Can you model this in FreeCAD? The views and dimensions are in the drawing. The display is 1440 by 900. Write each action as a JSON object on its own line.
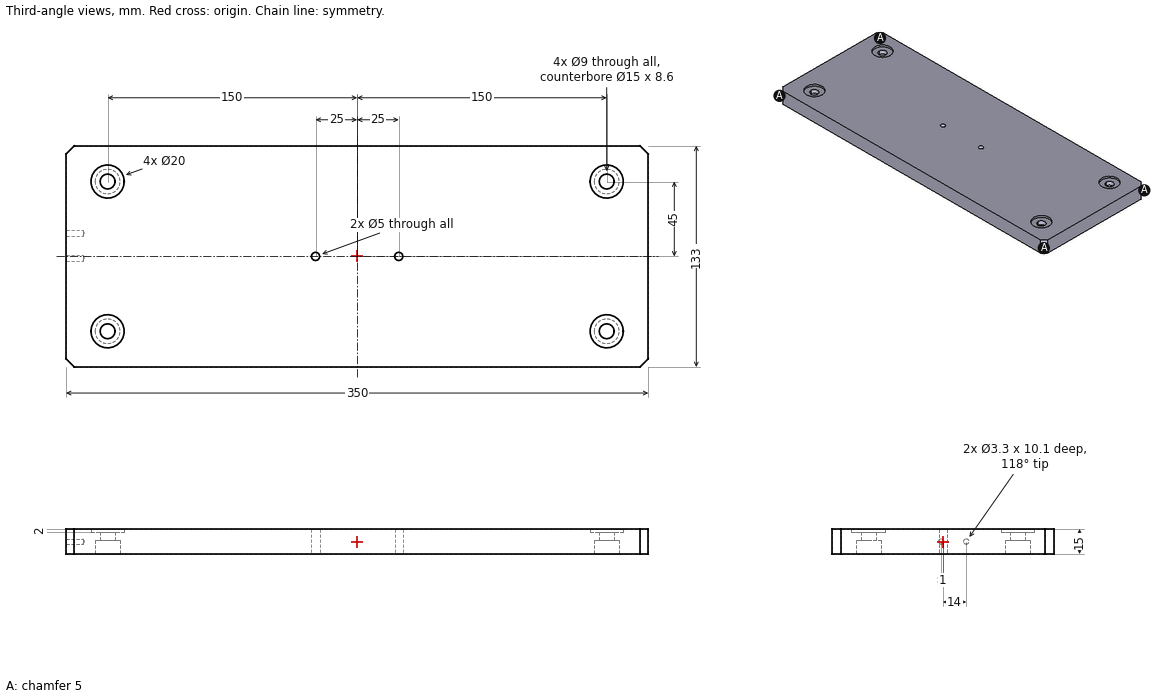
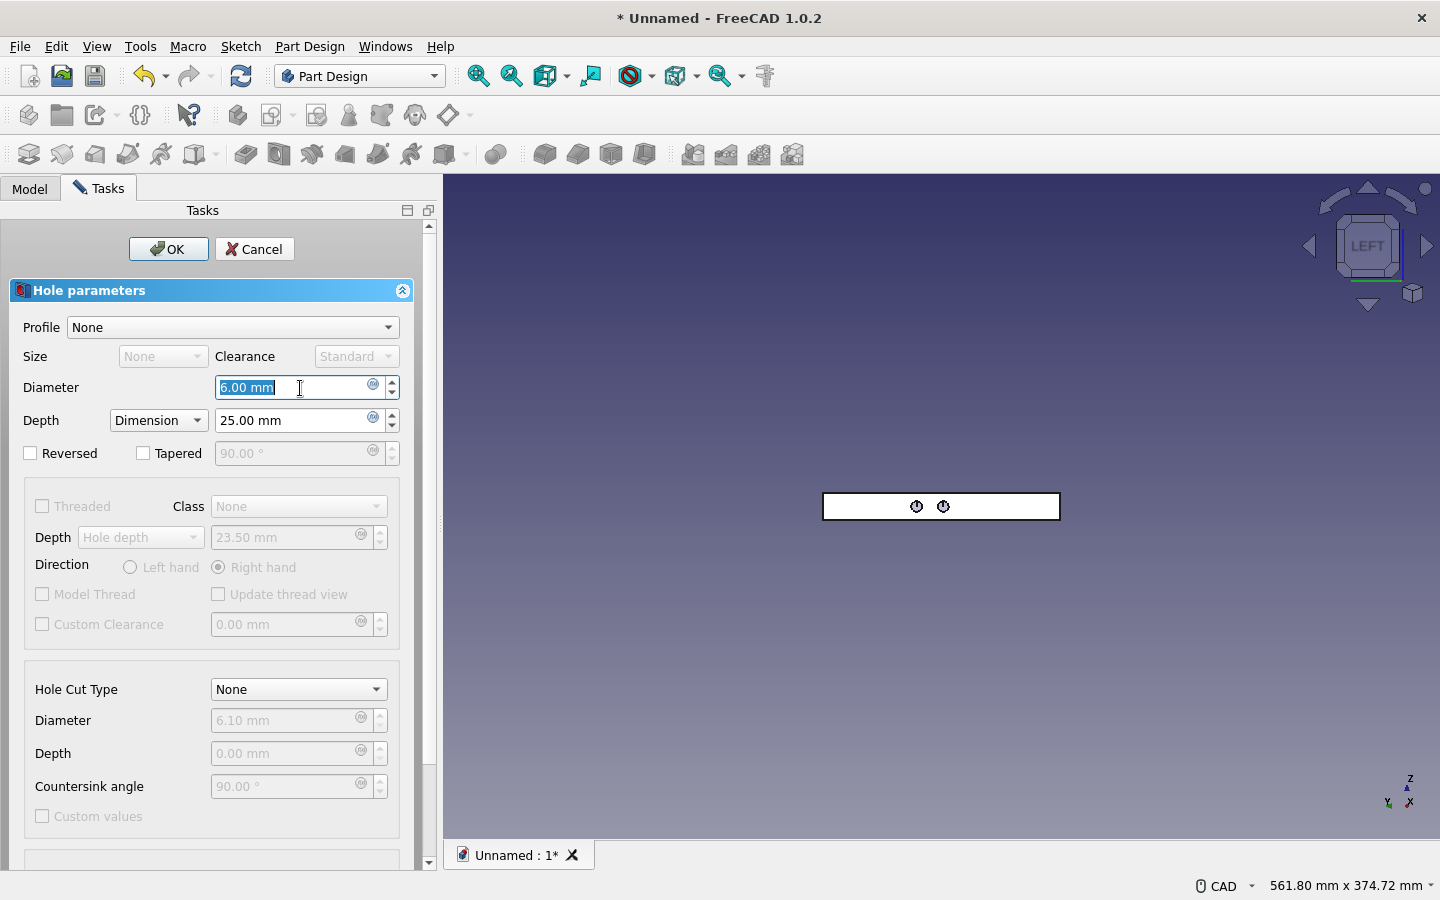
{"action": "type", "text": "3.3"}
{"action": "key", "text": "Tab"}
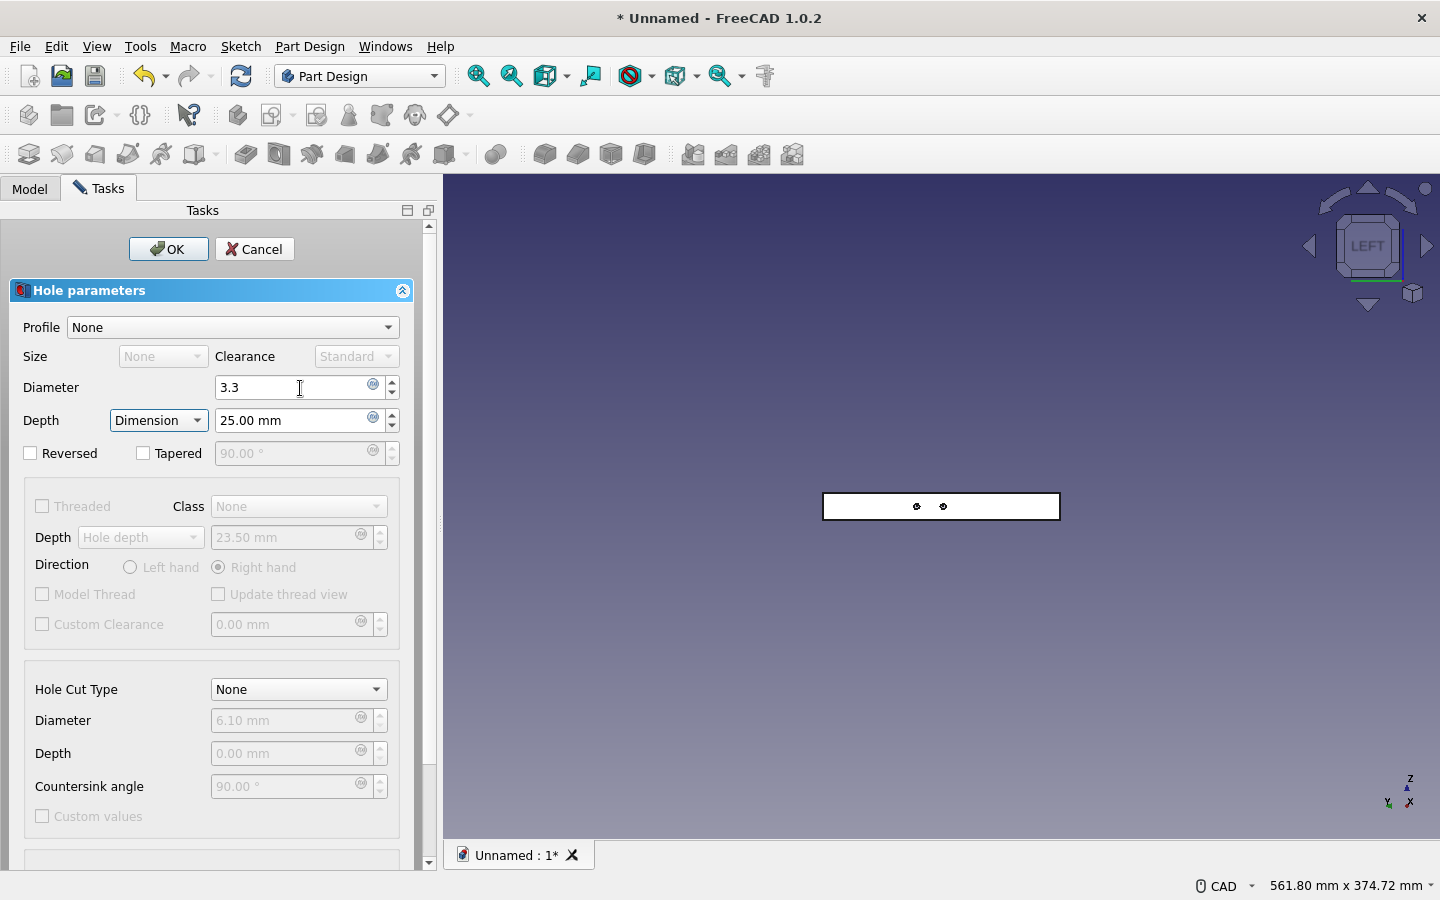
{"action": "triple_click", "coordinate": [300, 420]}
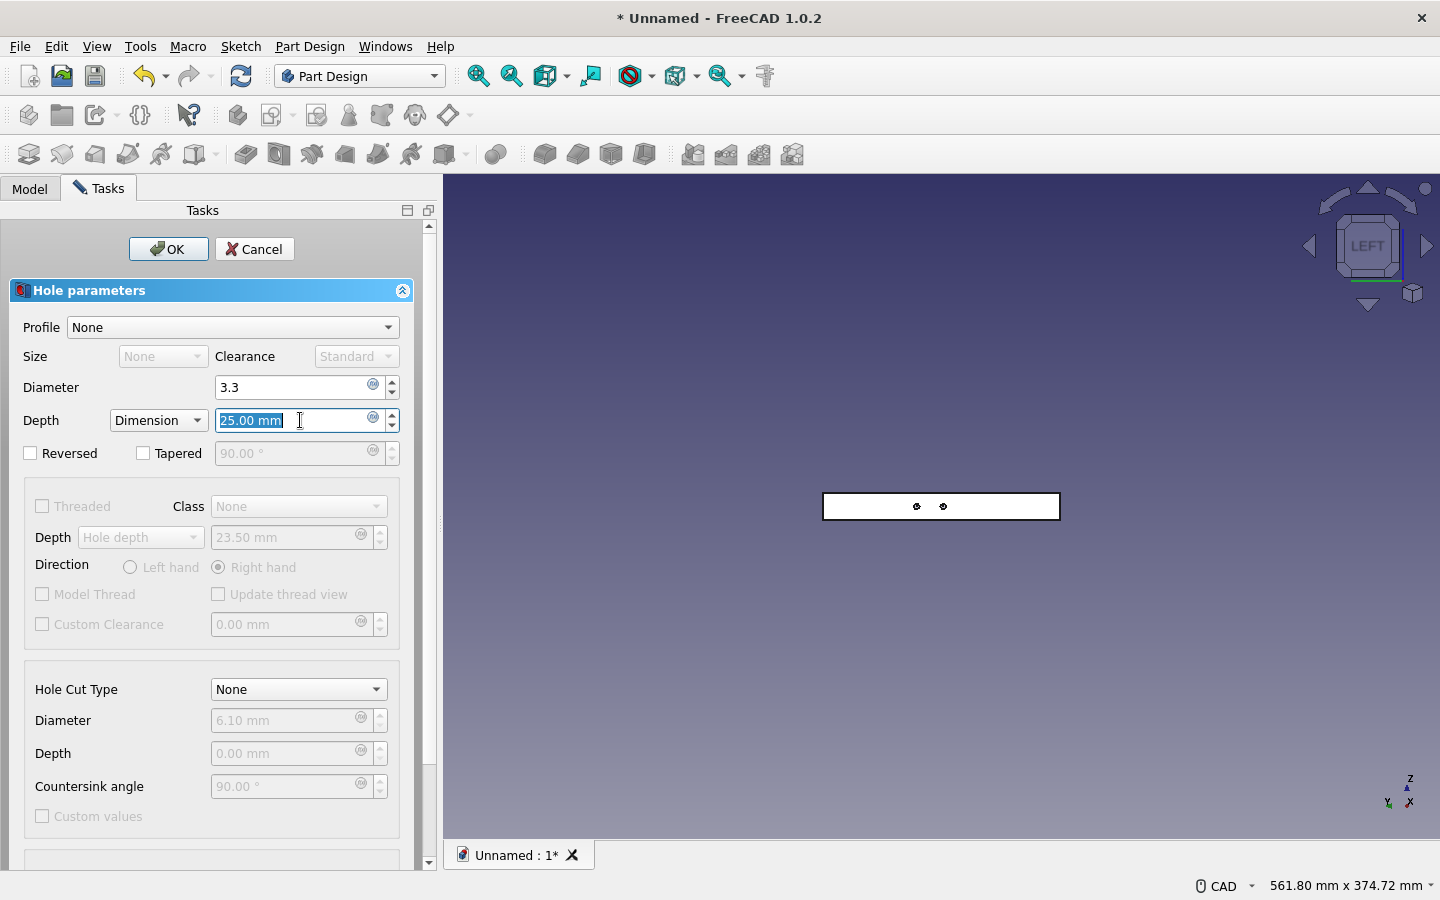
{"action": "type", "text": "10.1"}
{"action": "key", "text": "Tab"}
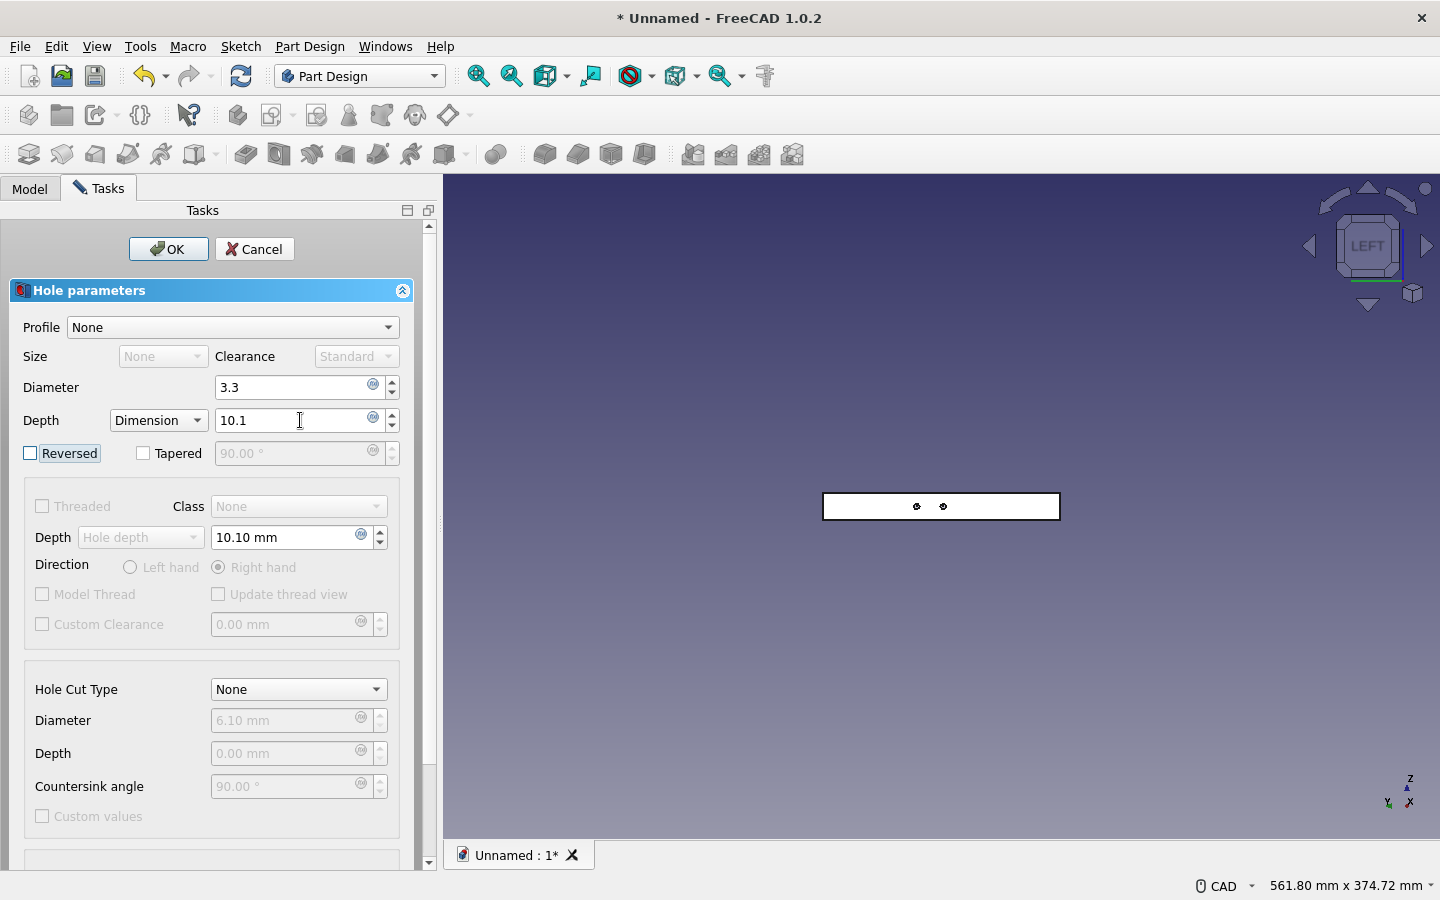
{"action": "left_click", "coordinate": [169, 249]}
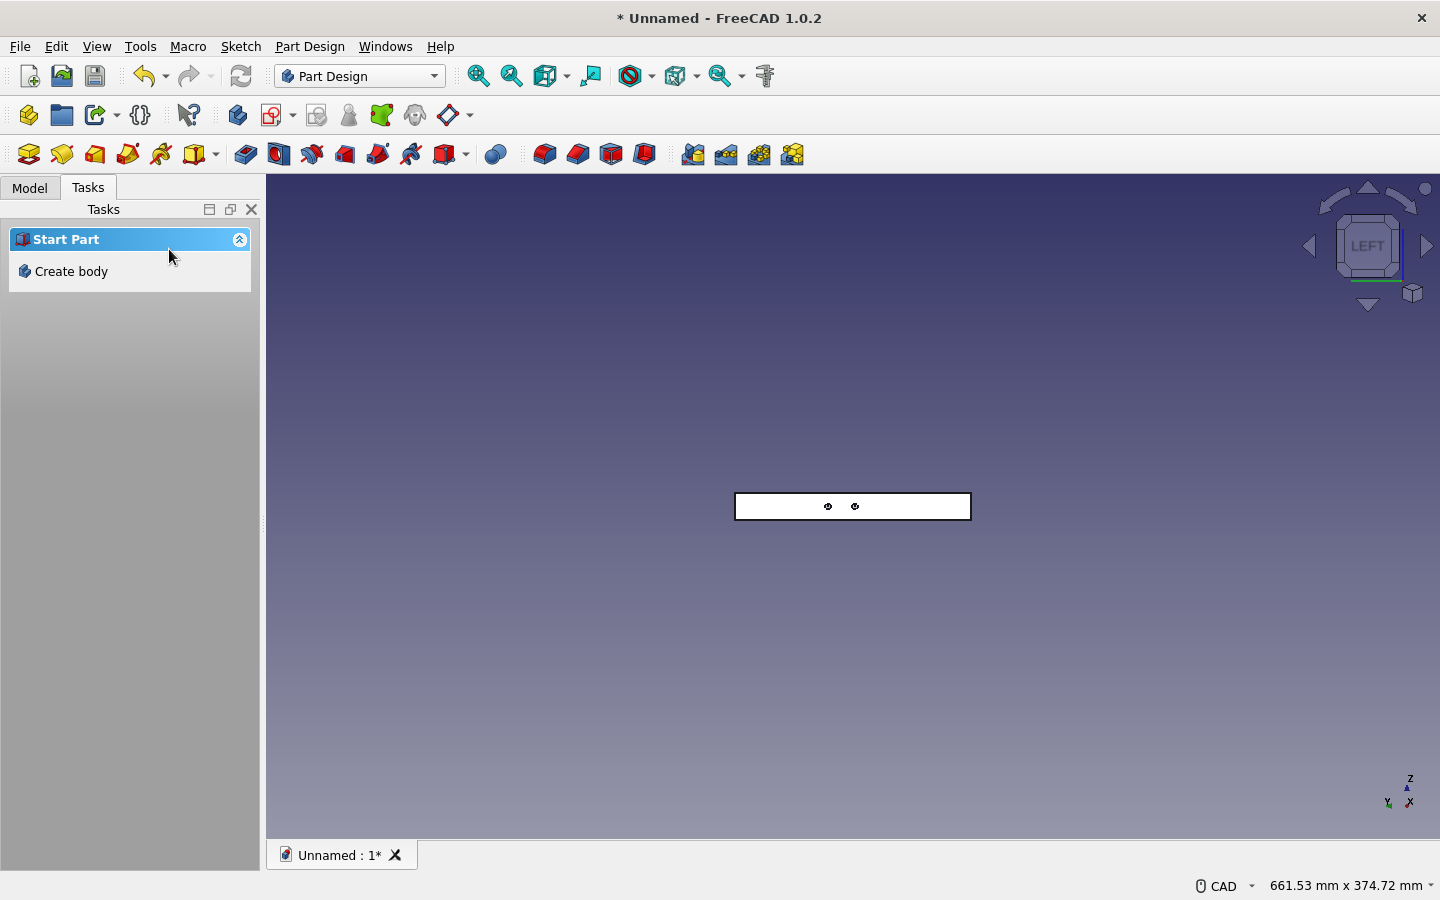
{"action": "key", "text": "v f"}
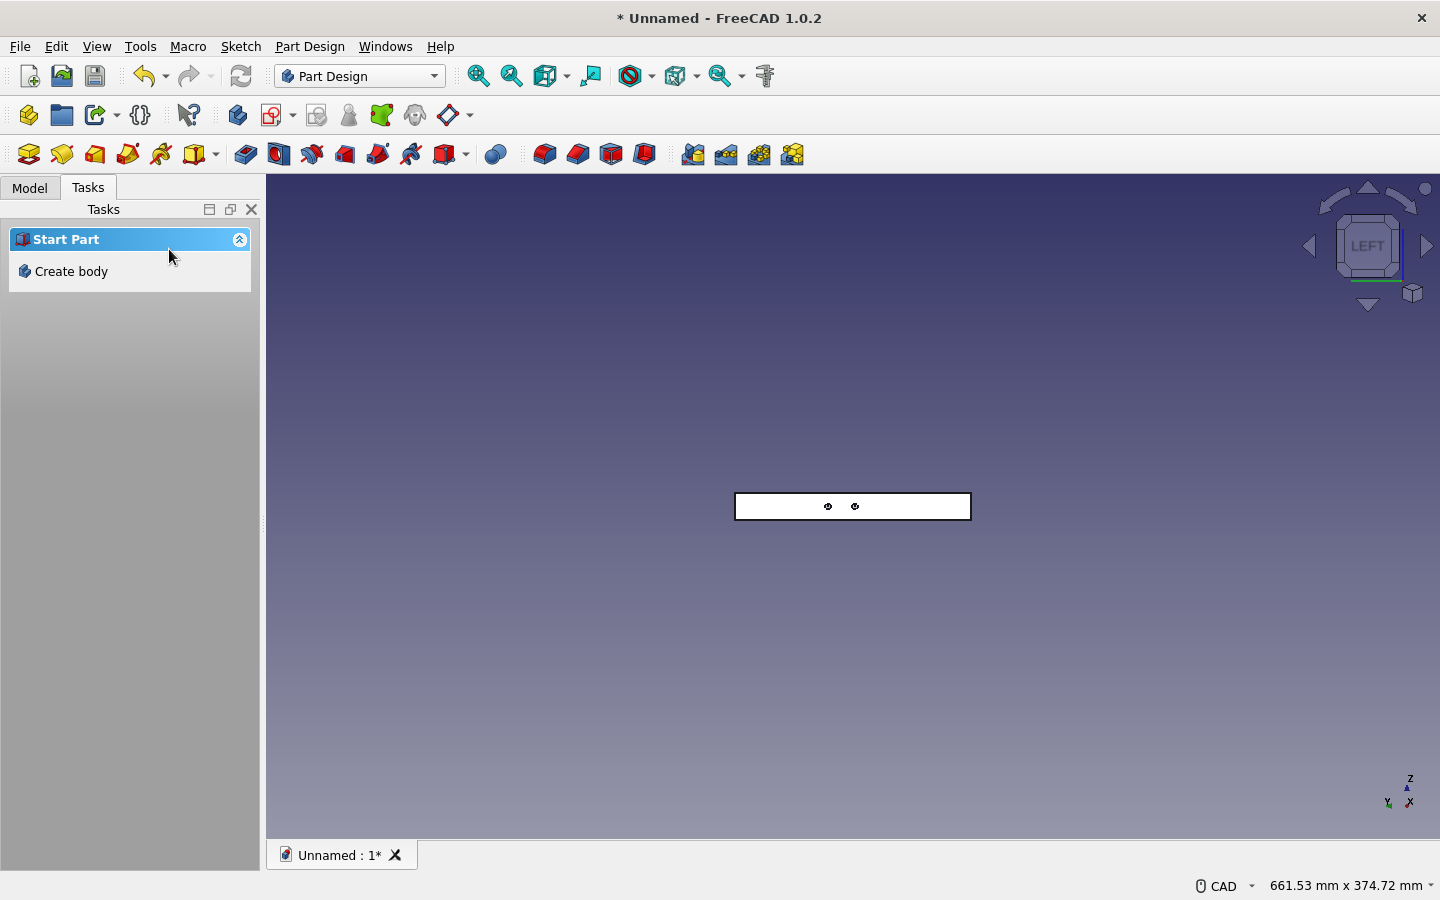
{"action": "left_click", "coordinate": [971, 505]}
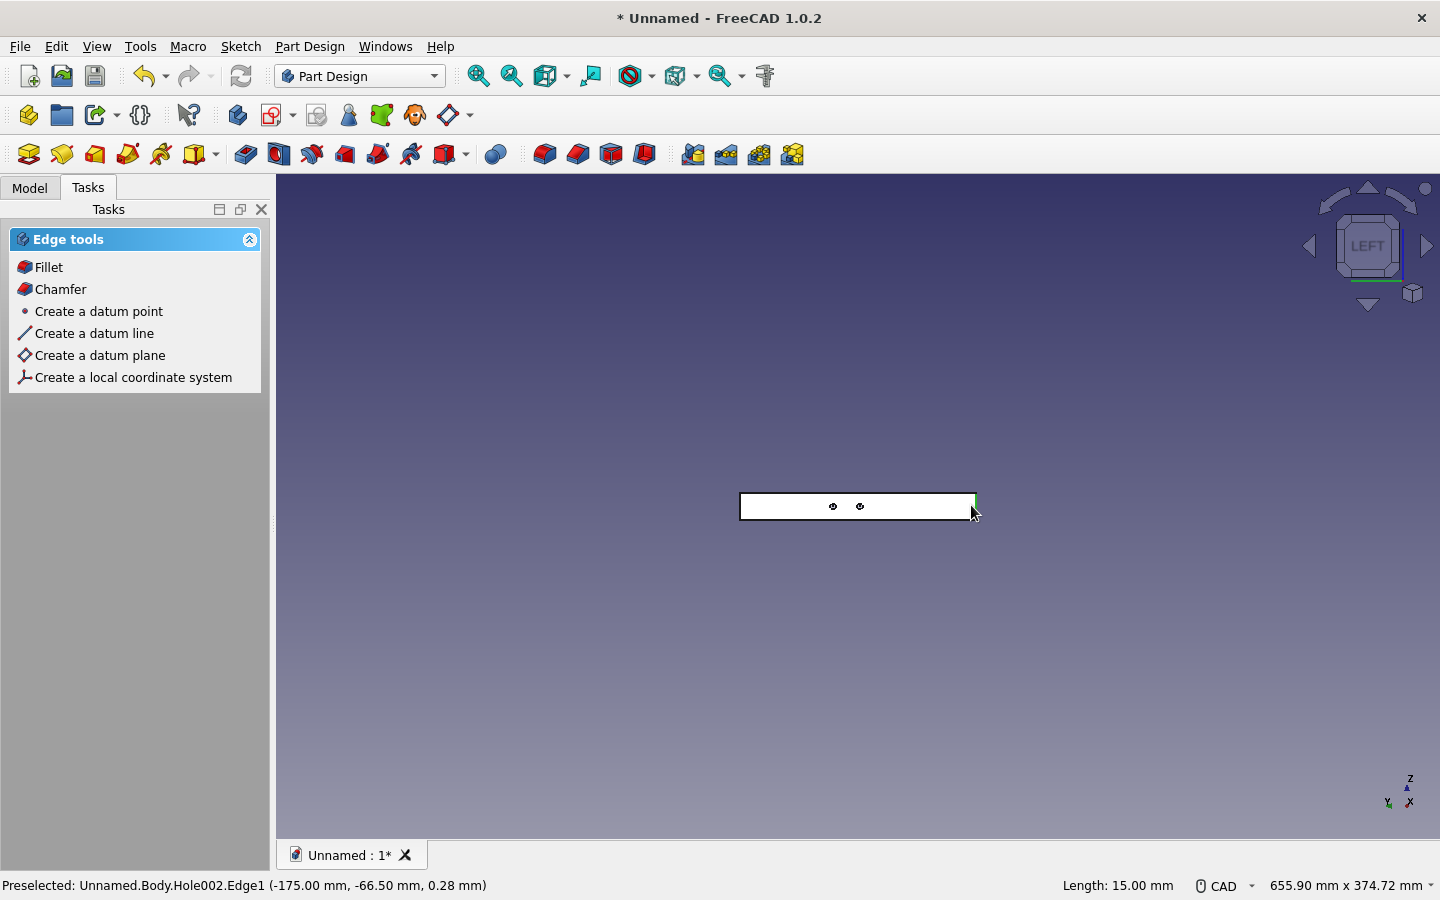
{"action": "left_click", "coordinate": [740, 505], "text": "ctrl"}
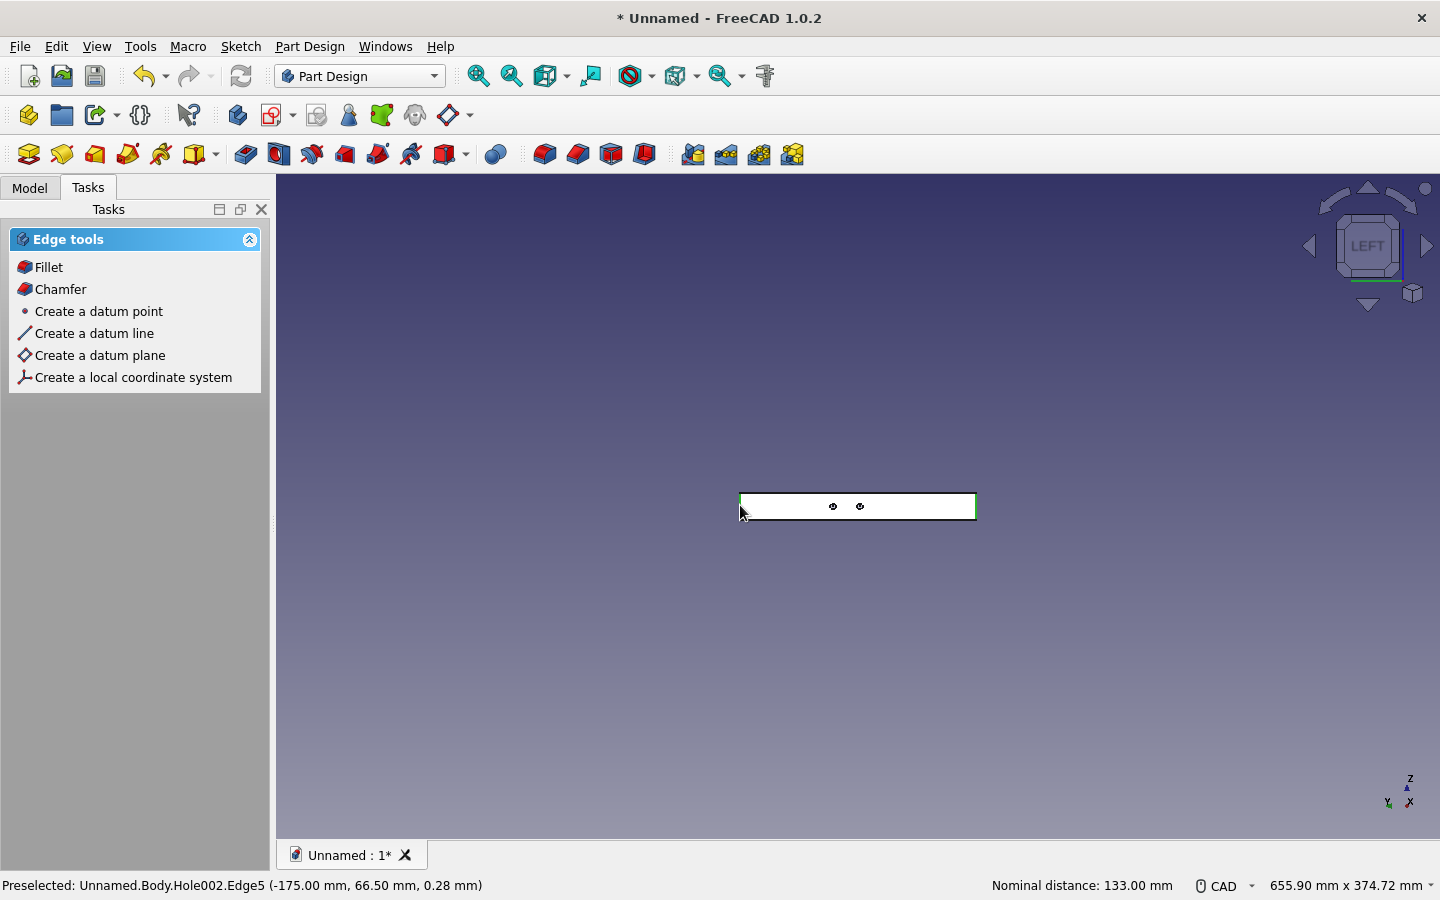
{"action": "key", "text": "0"}